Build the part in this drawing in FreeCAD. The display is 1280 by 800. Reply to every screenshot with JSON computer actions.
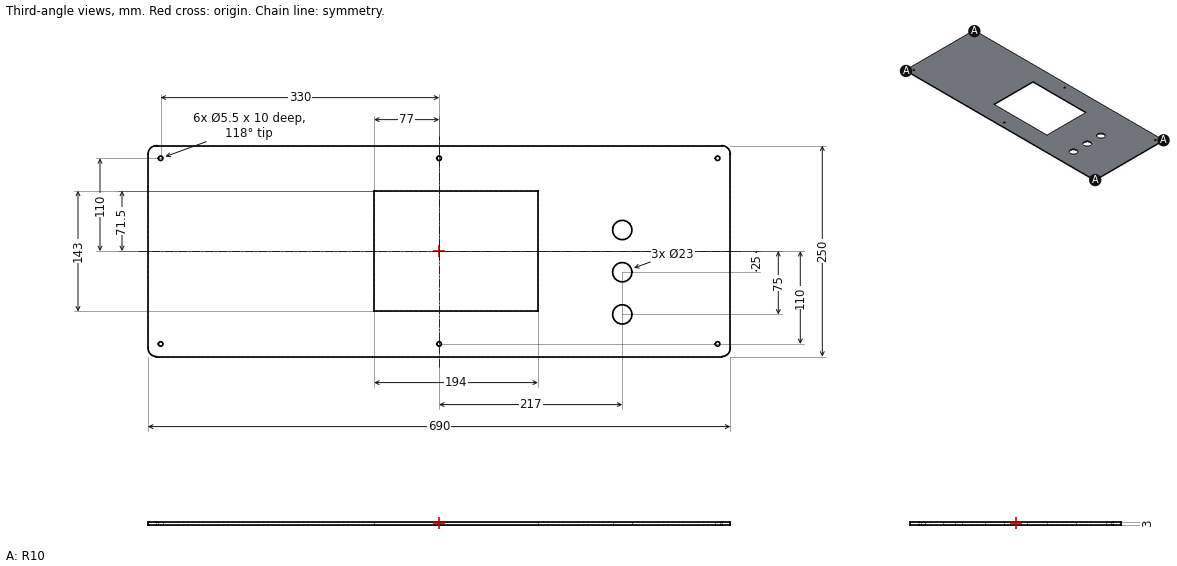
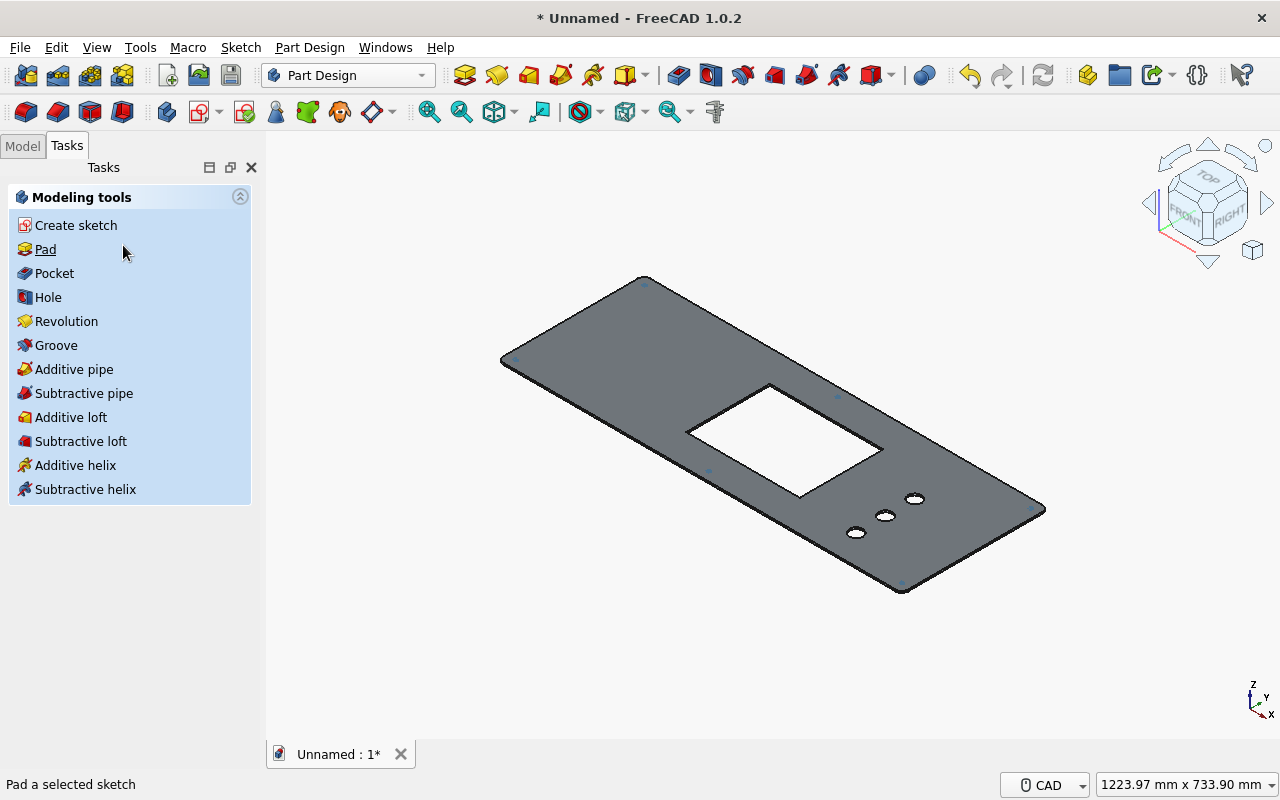
{"action": "left_click", "coordinate": [712, 76]}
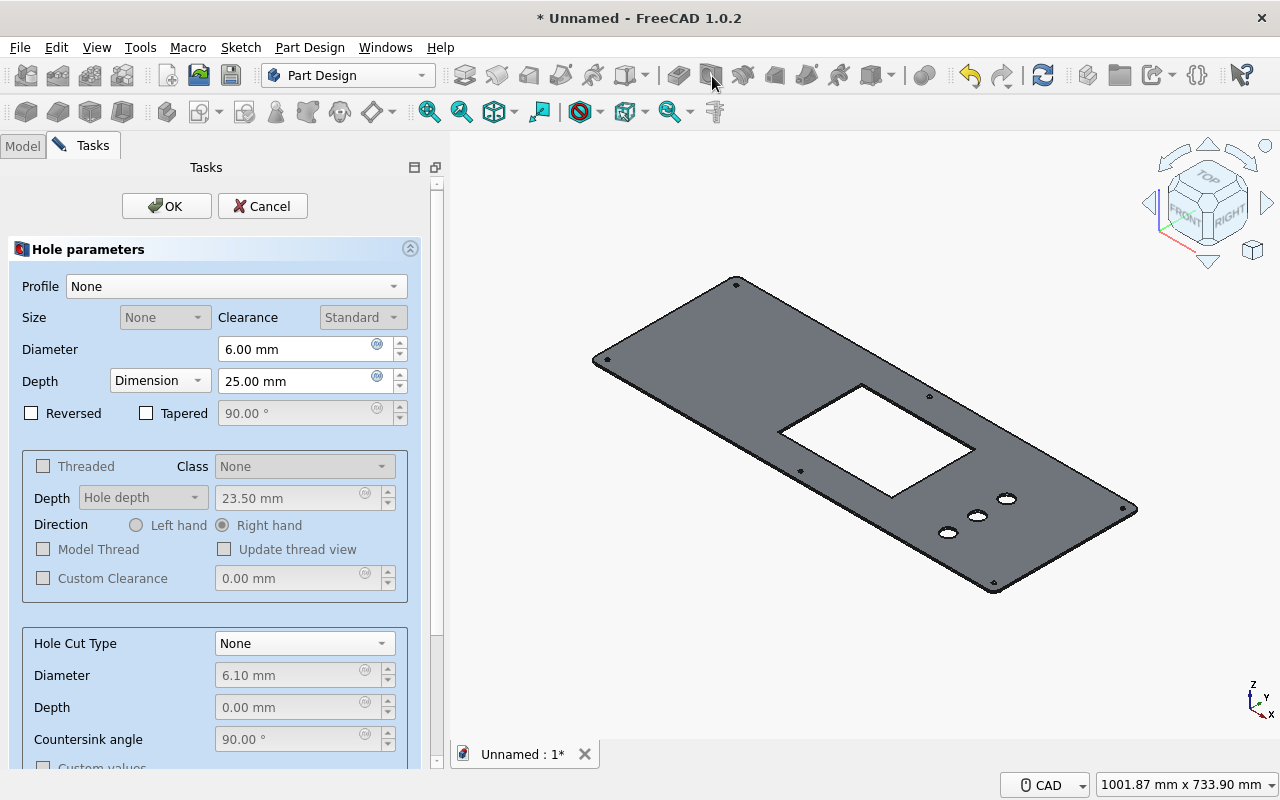
{"action": "triple_click", "coordinate": [305, 349]}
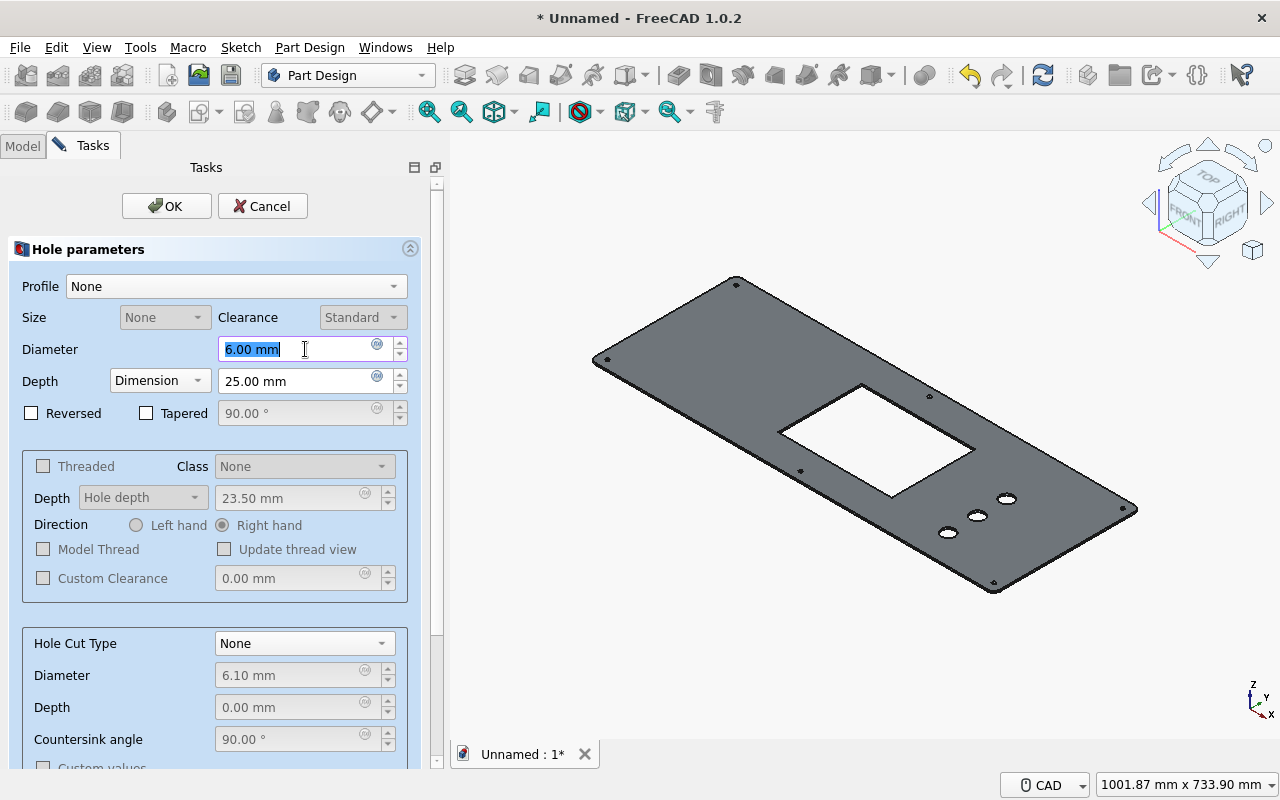
{"action": "type", "text": "5.5"}
{"action": "key", "text": "Tab"}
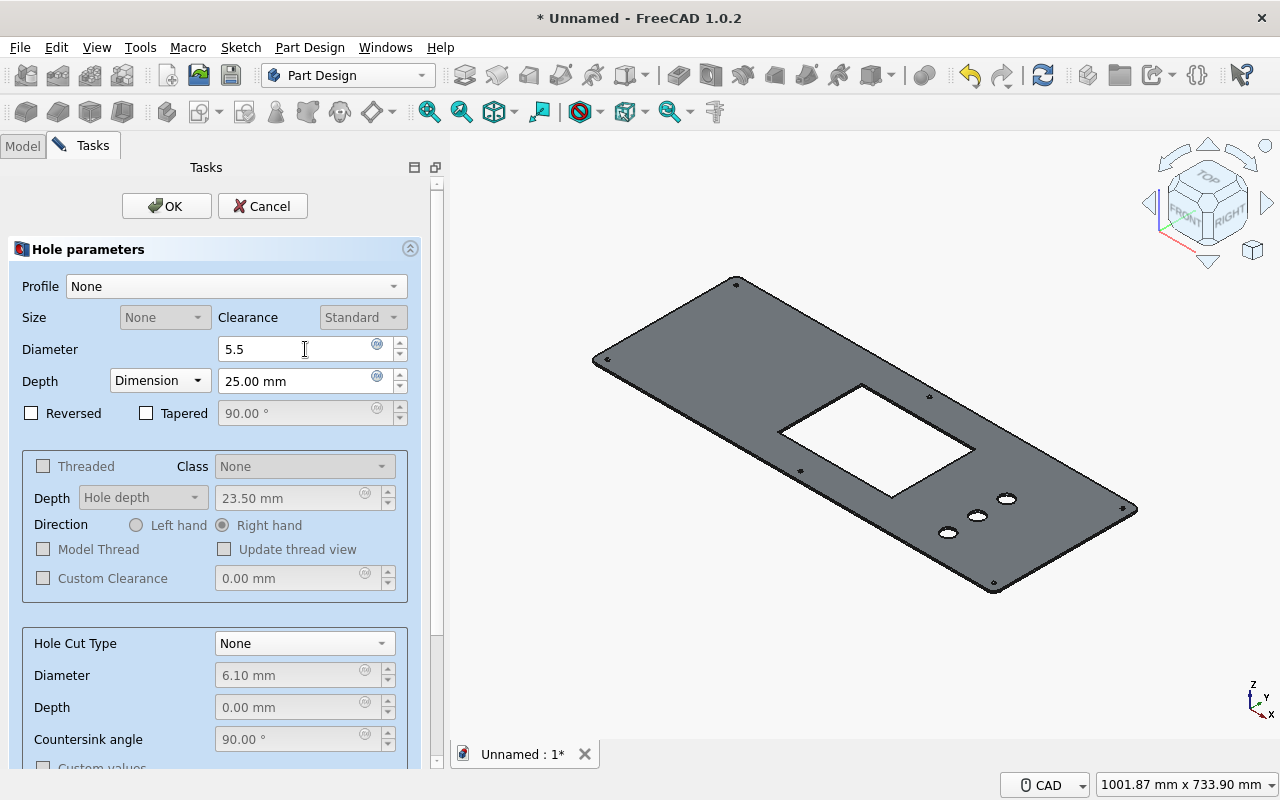
{"action": "triple_click", "coordinate": [305, 381]}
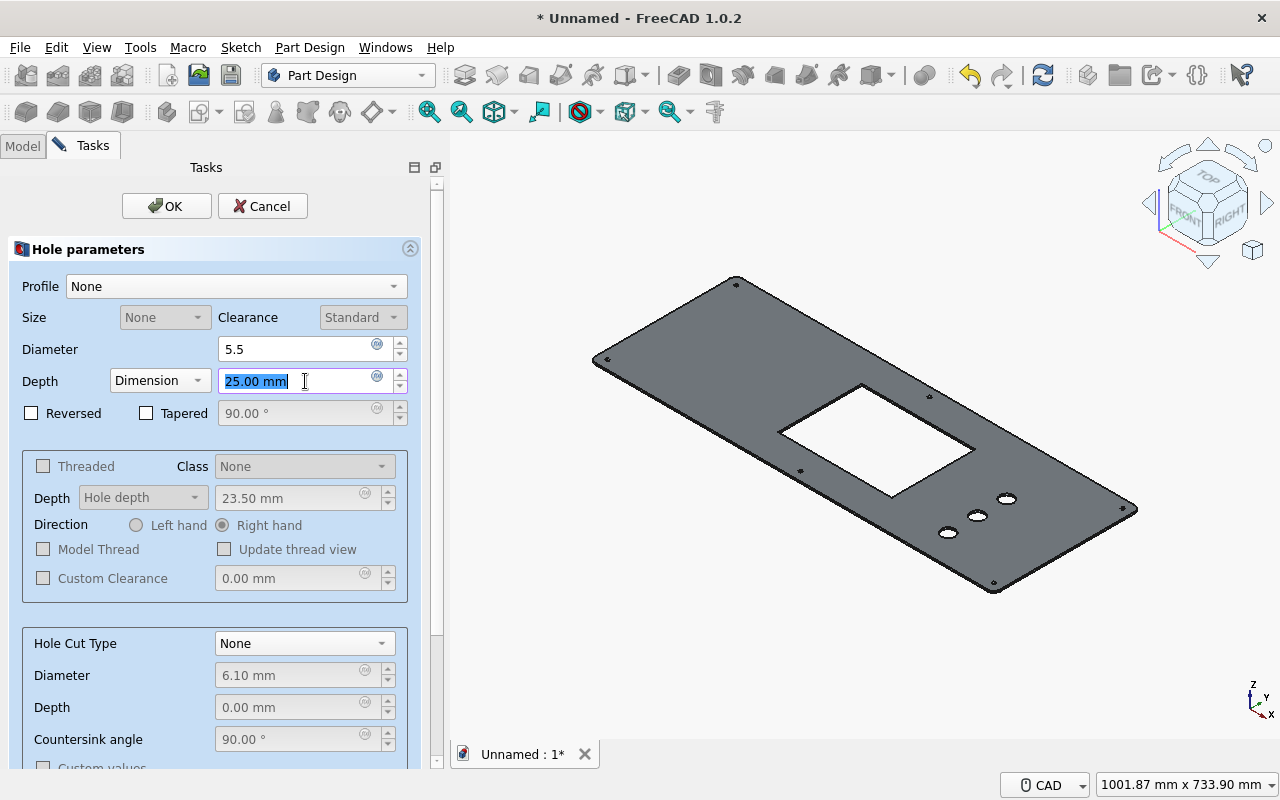
{"action": "type", "text": "10"}
{"action": "key", "text": "Tab"}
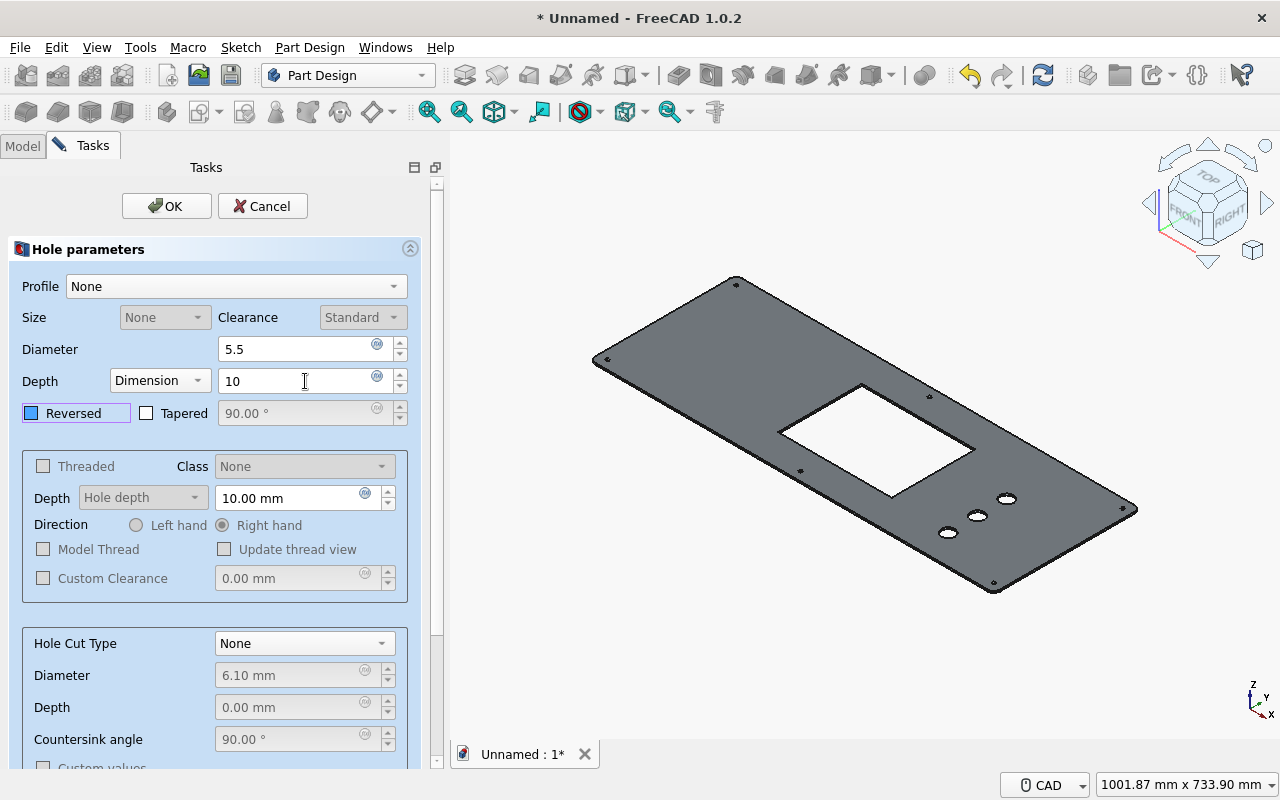
{"action": "left_click", "coordinate": [167, 206]}